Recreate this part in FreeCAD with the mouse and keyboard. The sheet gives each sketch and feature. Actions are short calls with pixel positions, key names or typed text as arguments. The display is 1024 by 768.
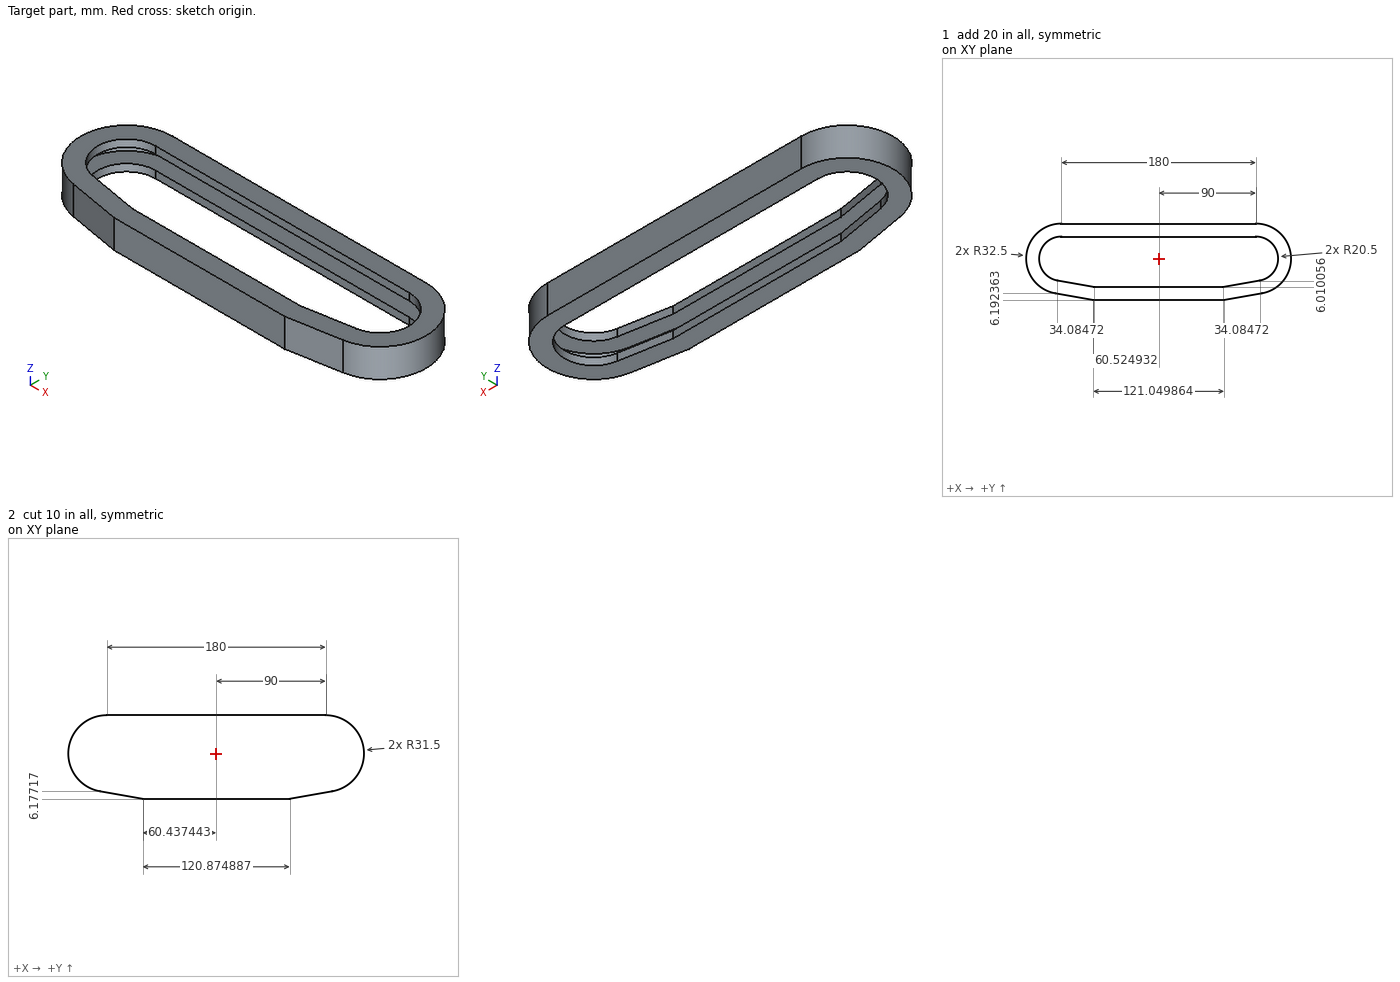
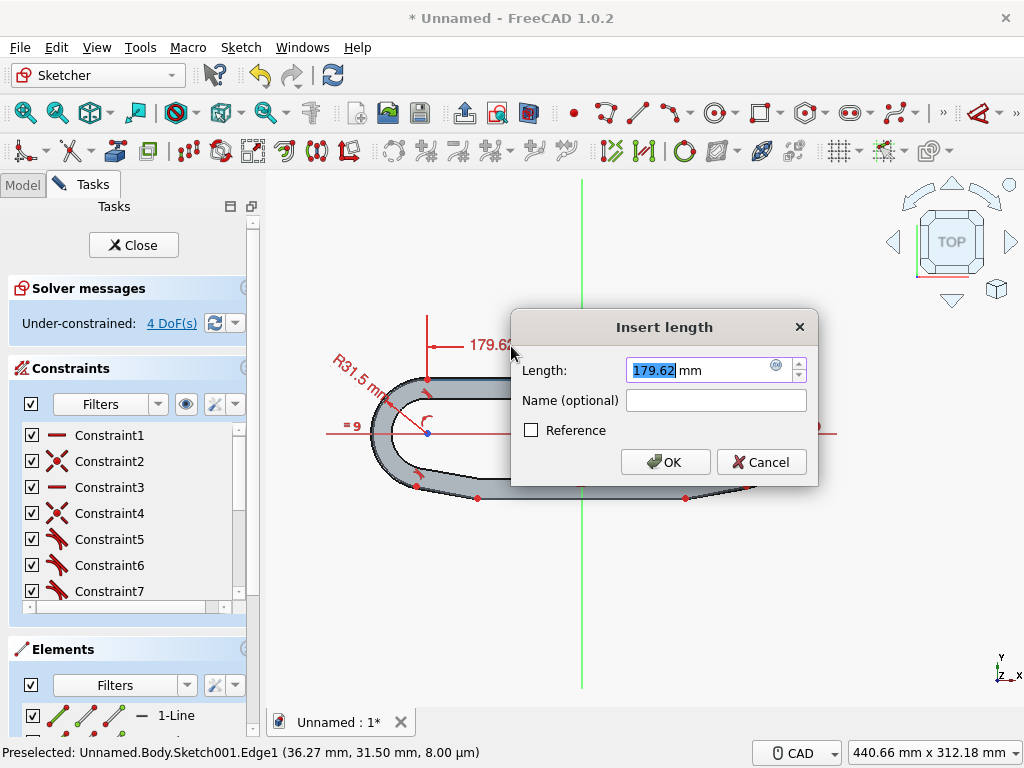
text(180)
key(Return)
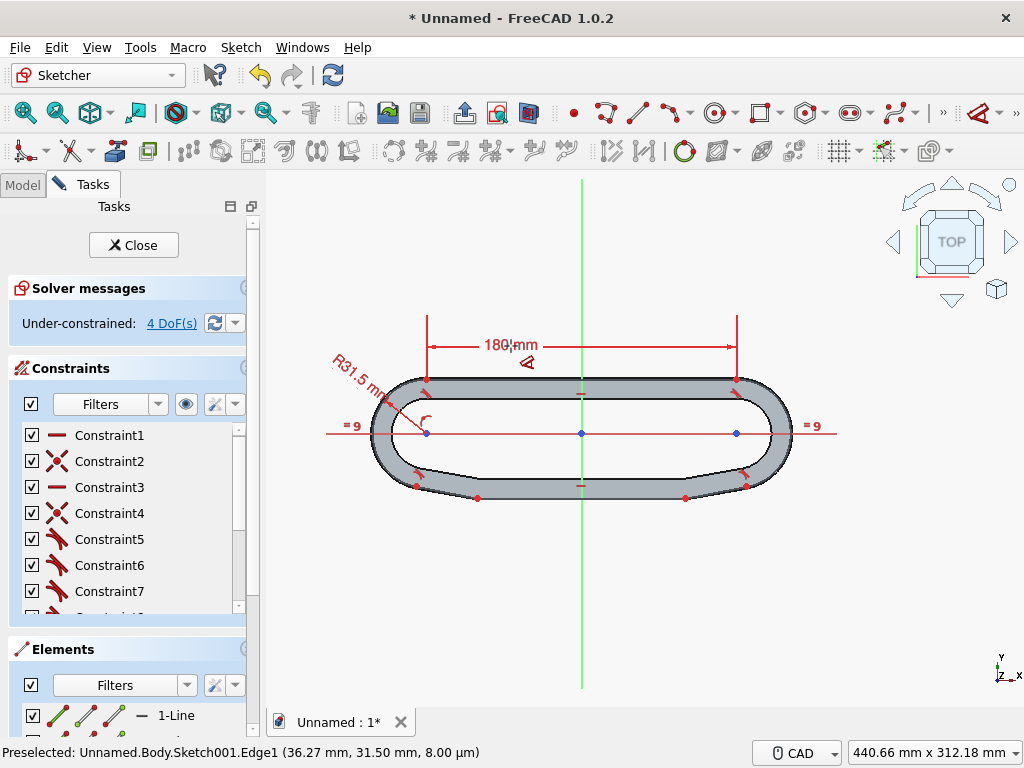
click(737, 380)
click(659, 346)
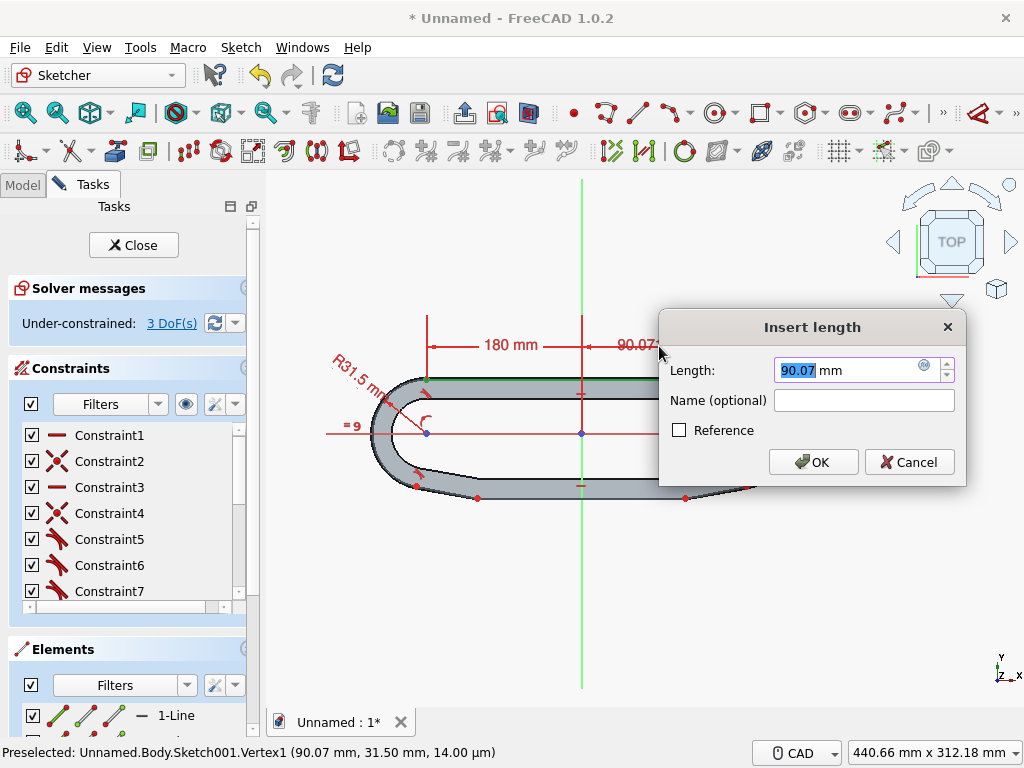
text(90)
key(Return)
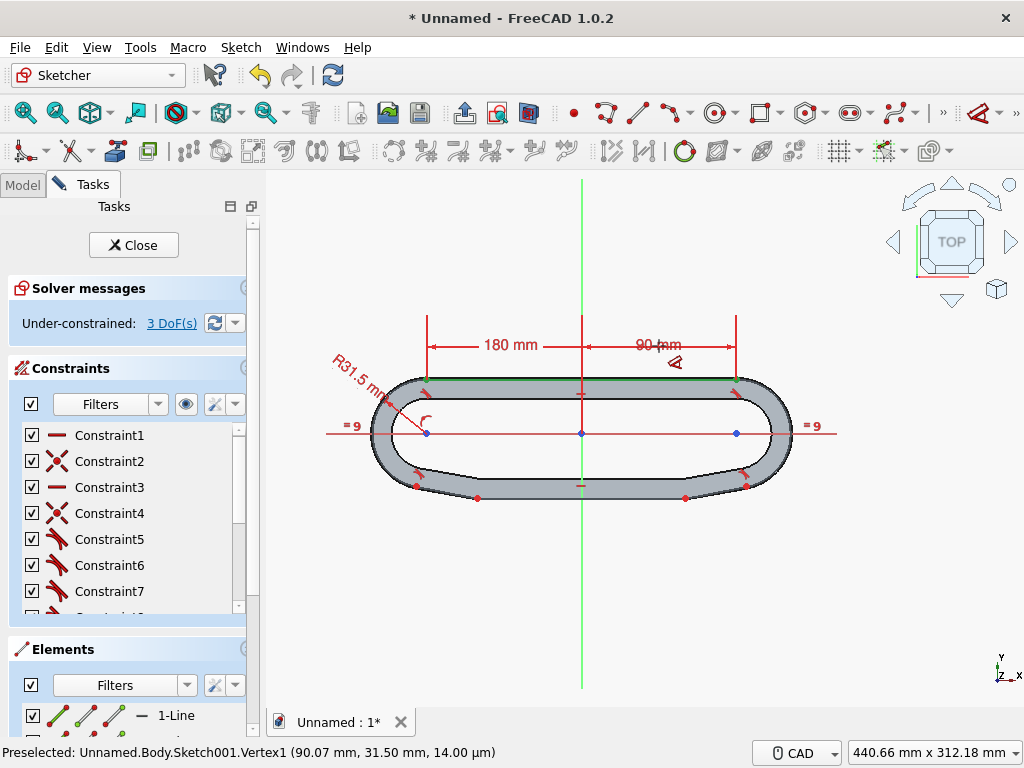
scroll(435, 491, up, 7)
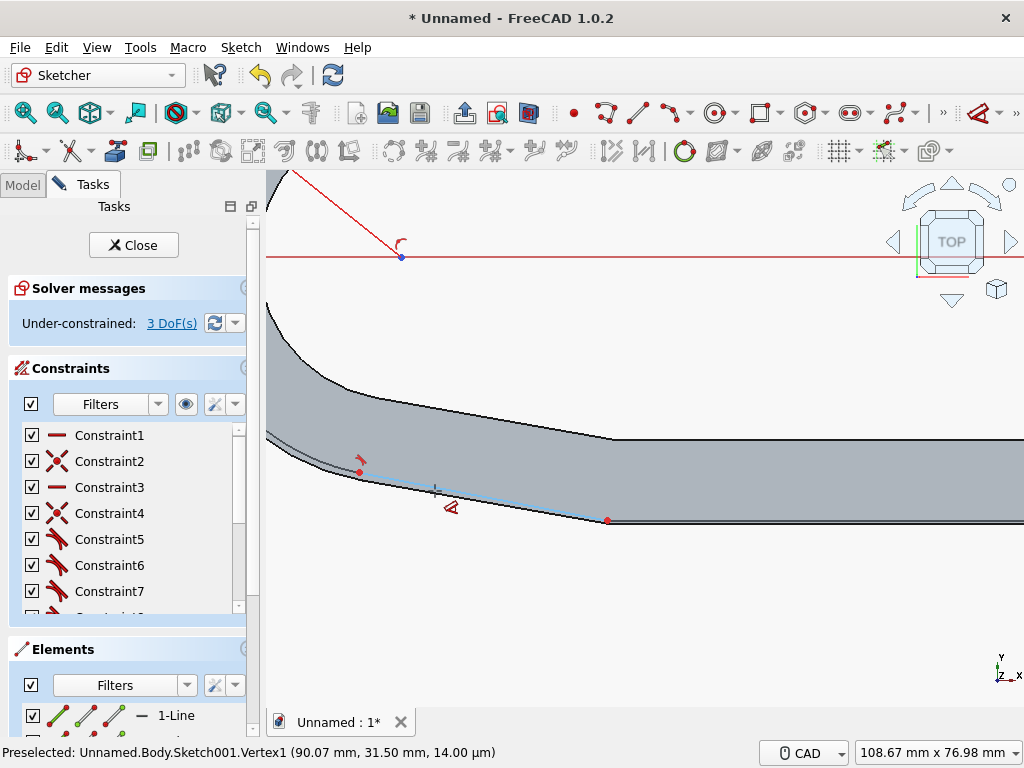
click(434, 487)
click(325, 497)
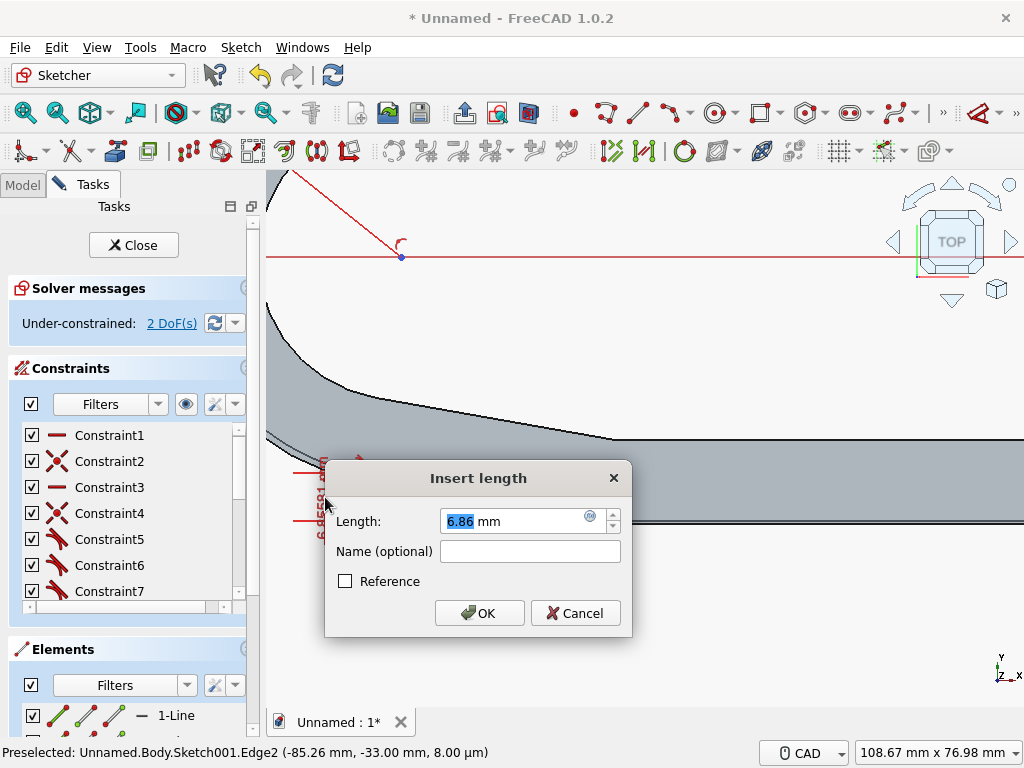
text(6.17717)
key(Return)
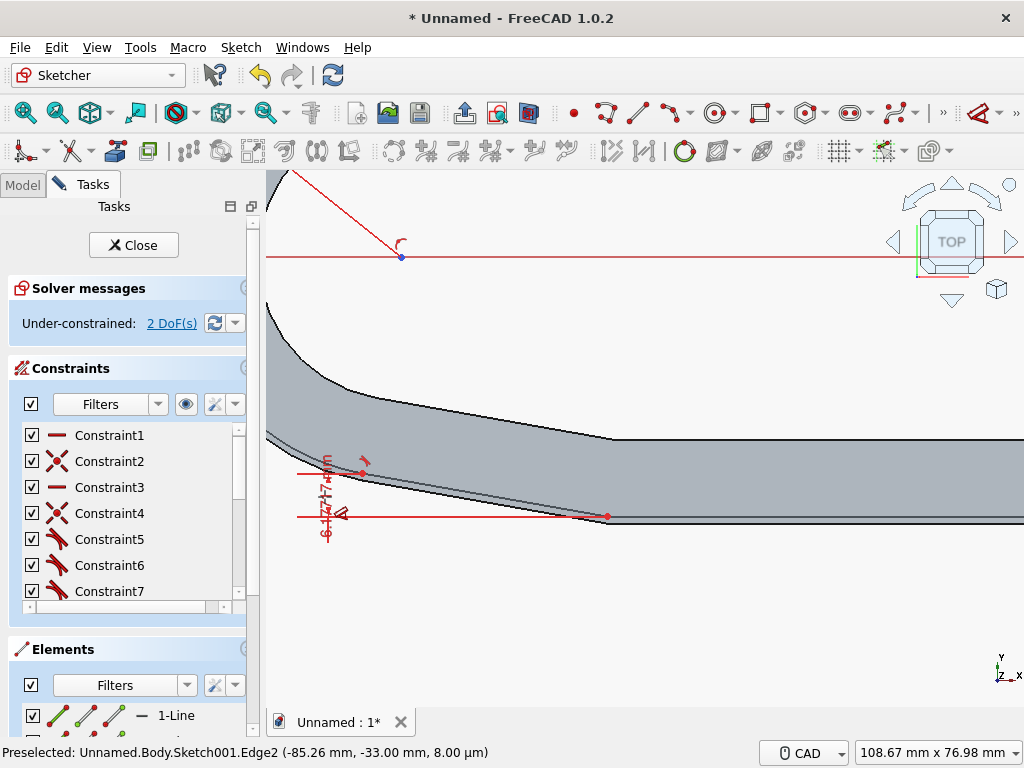
scroll(428, 491, down, 7)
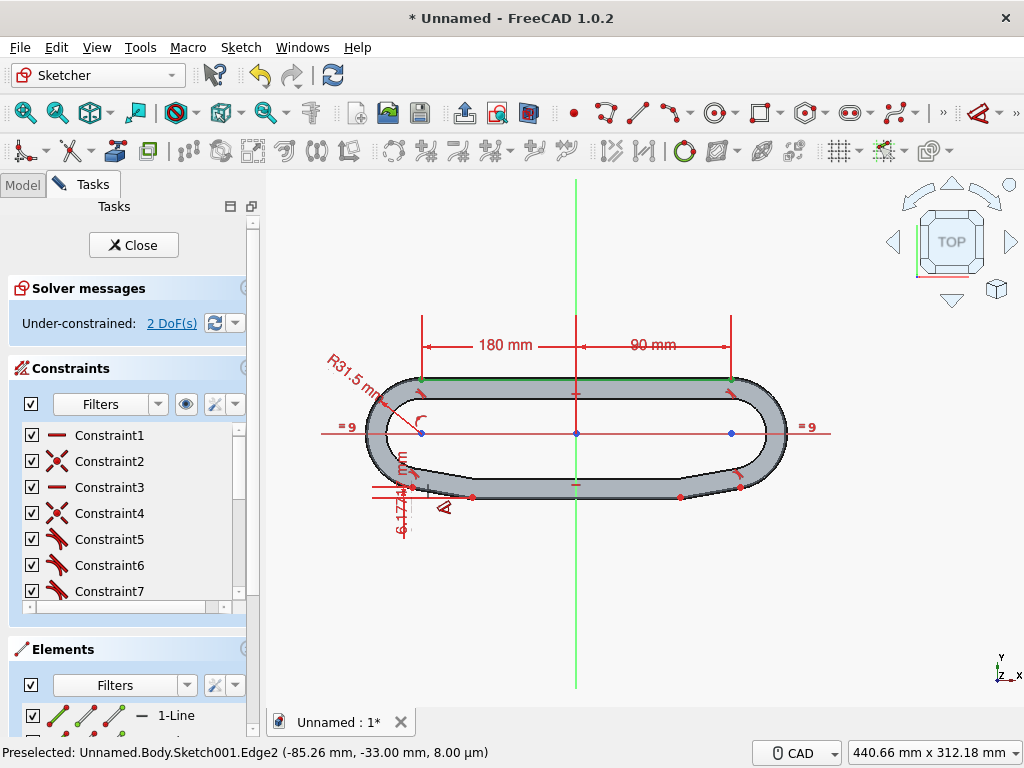
click(514, 498)
click(529, 532)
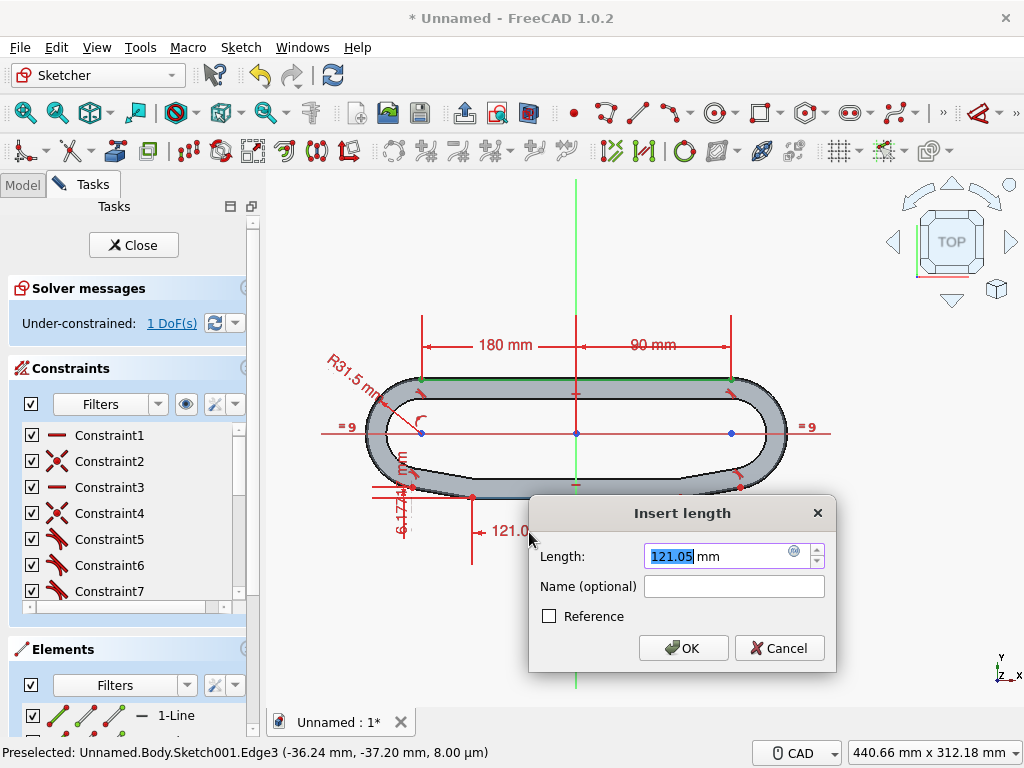
text(120.874887)
key(Return)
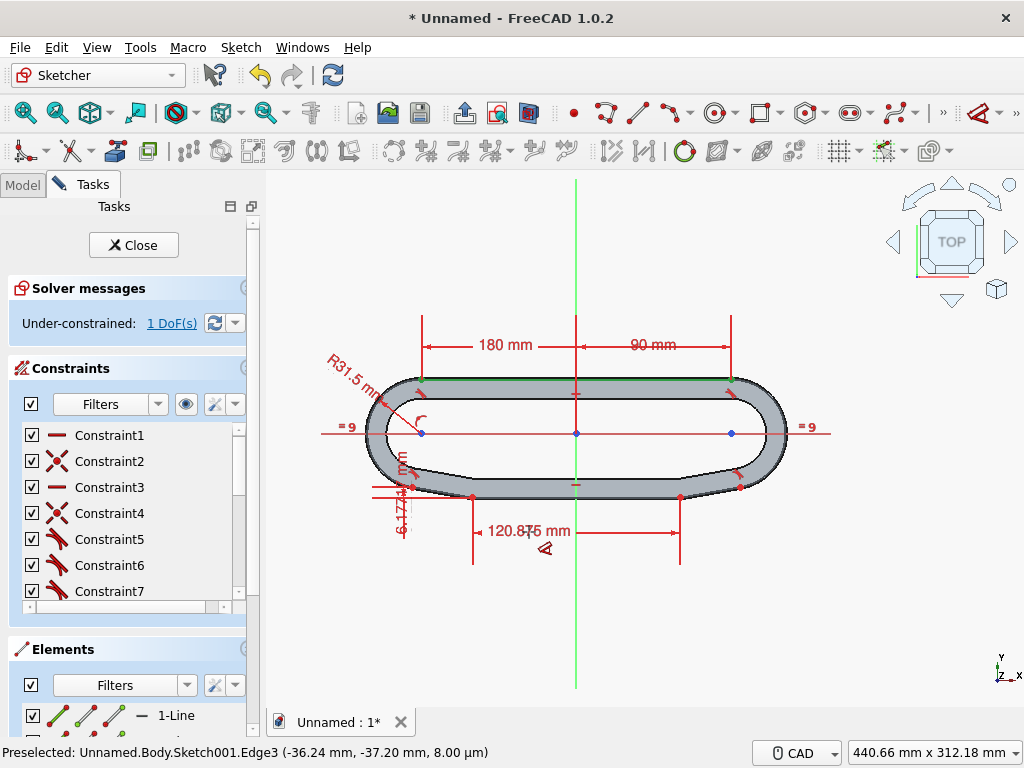
click(473, 498)
click(524, 400)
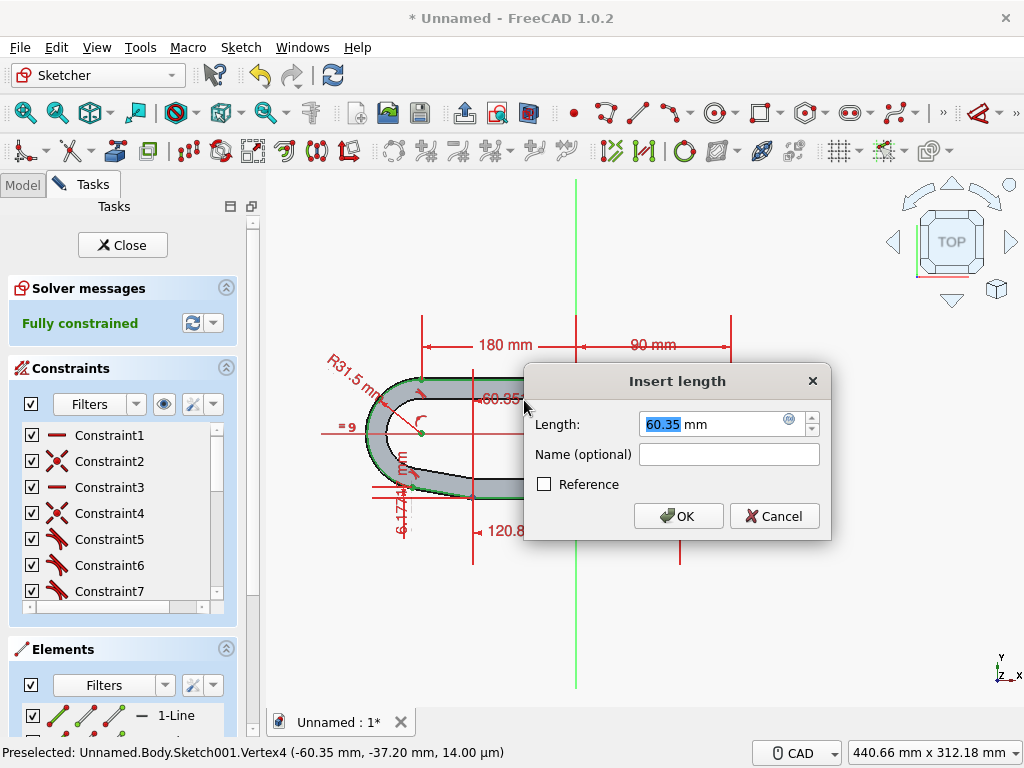
text(60.437443)
key(Return)
key(Escape)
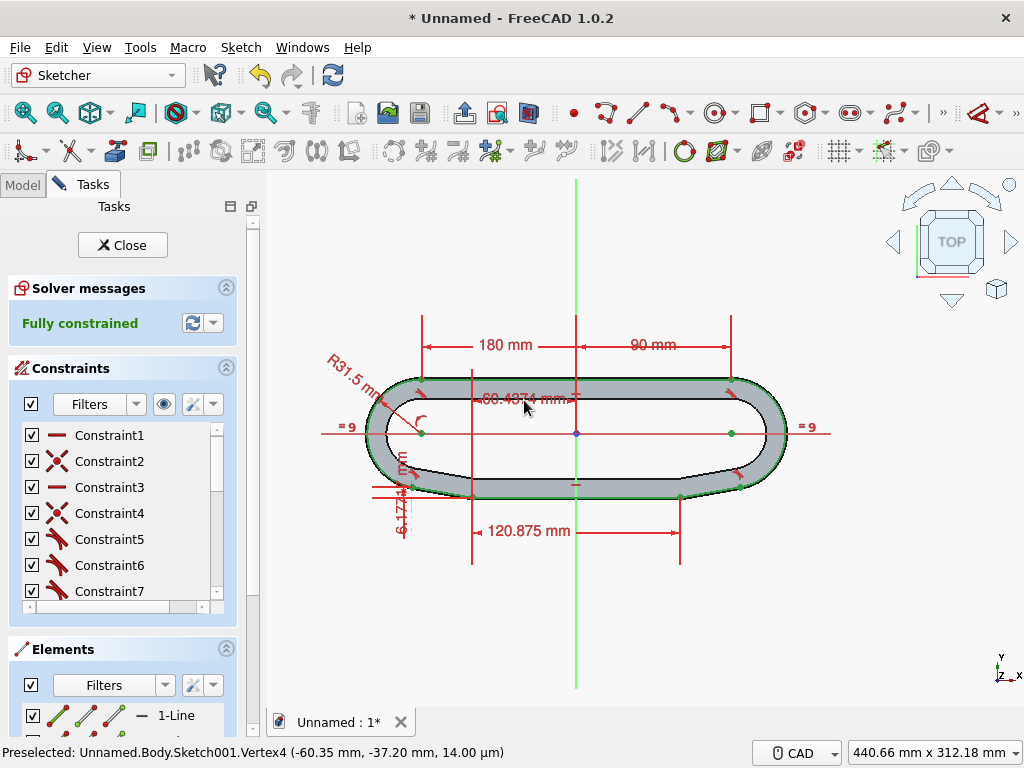
click(123, 245)